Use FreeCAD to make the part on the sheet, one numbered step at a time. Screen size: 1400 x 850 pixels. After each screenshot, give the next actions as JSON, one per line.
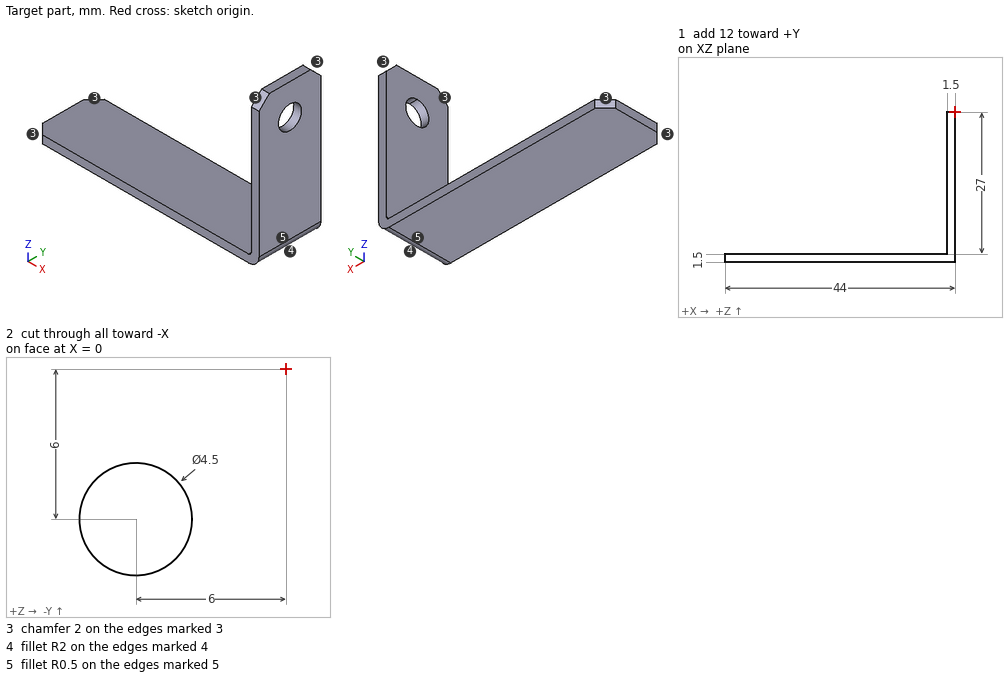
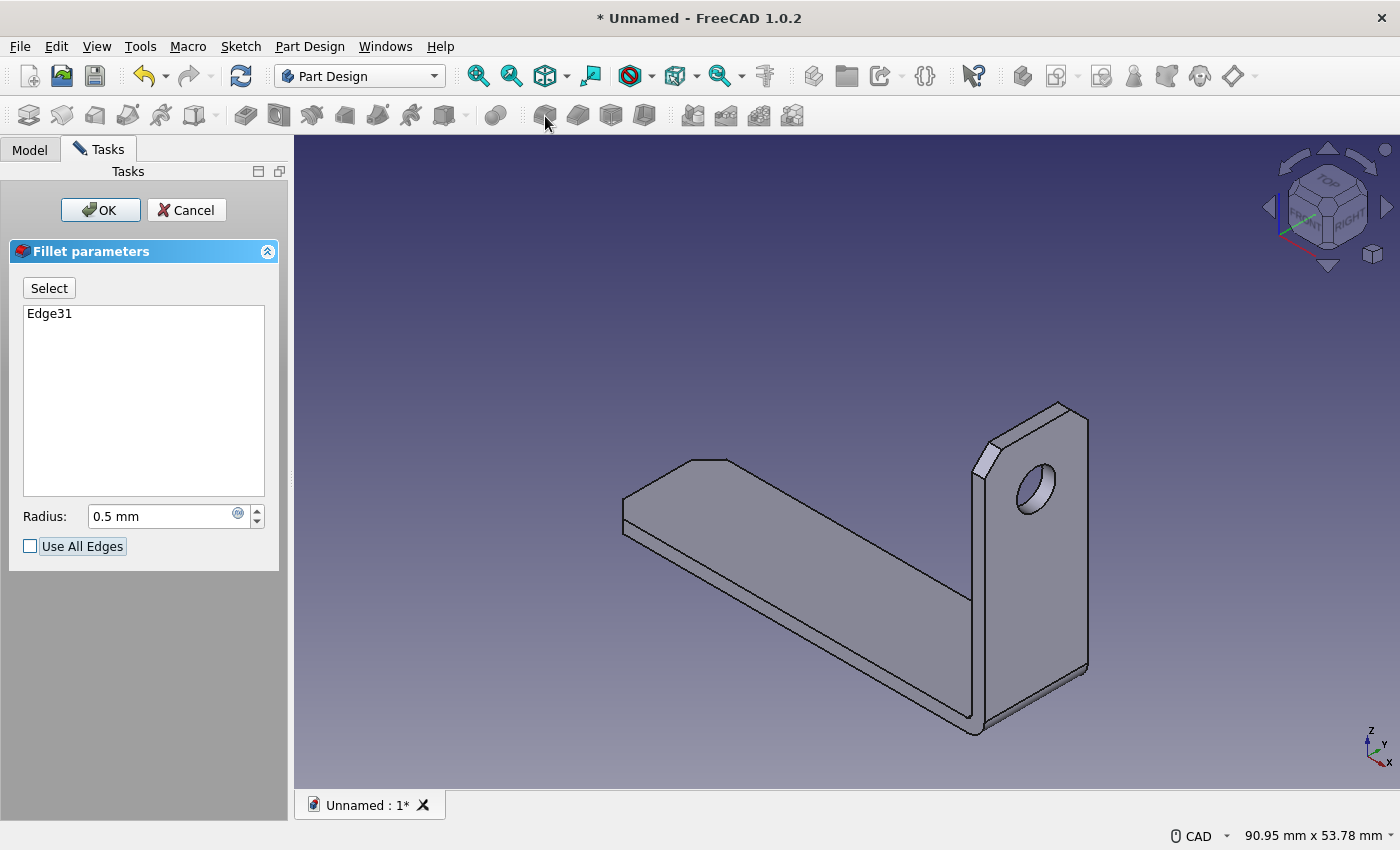
{"action": "left_click", "coordinate": [101, 210]}